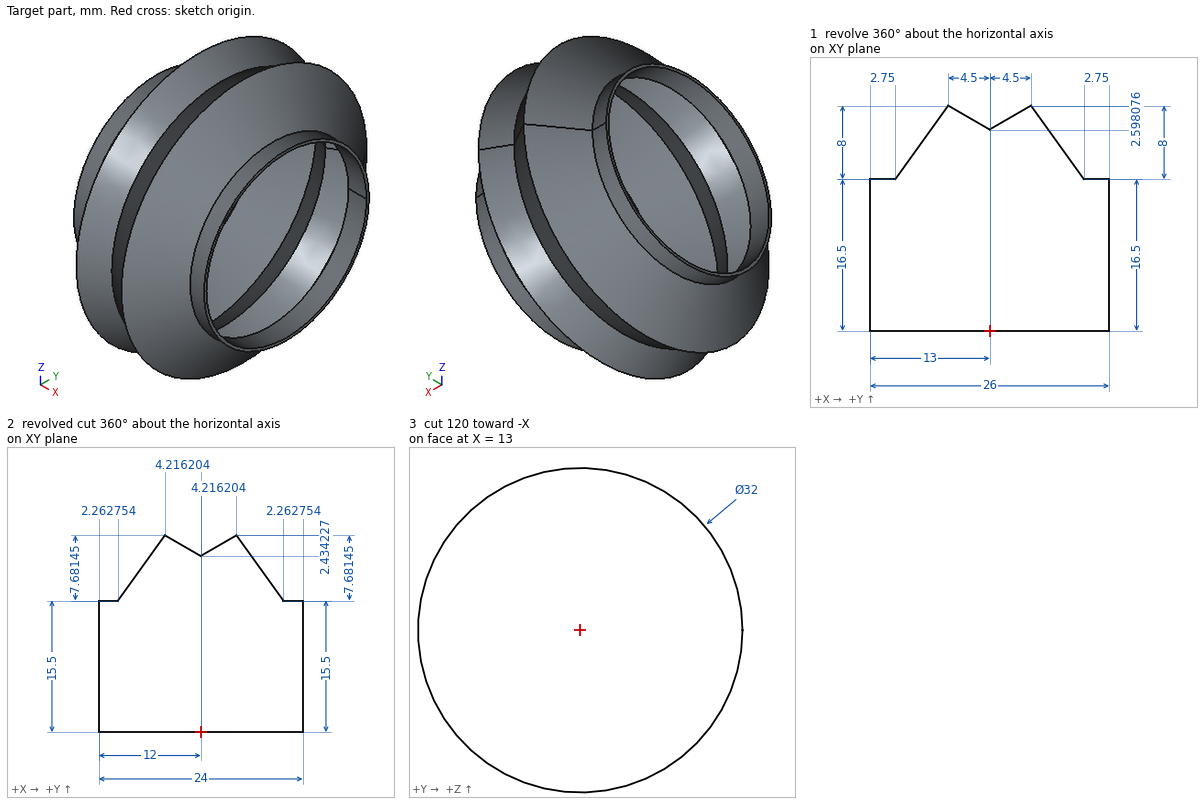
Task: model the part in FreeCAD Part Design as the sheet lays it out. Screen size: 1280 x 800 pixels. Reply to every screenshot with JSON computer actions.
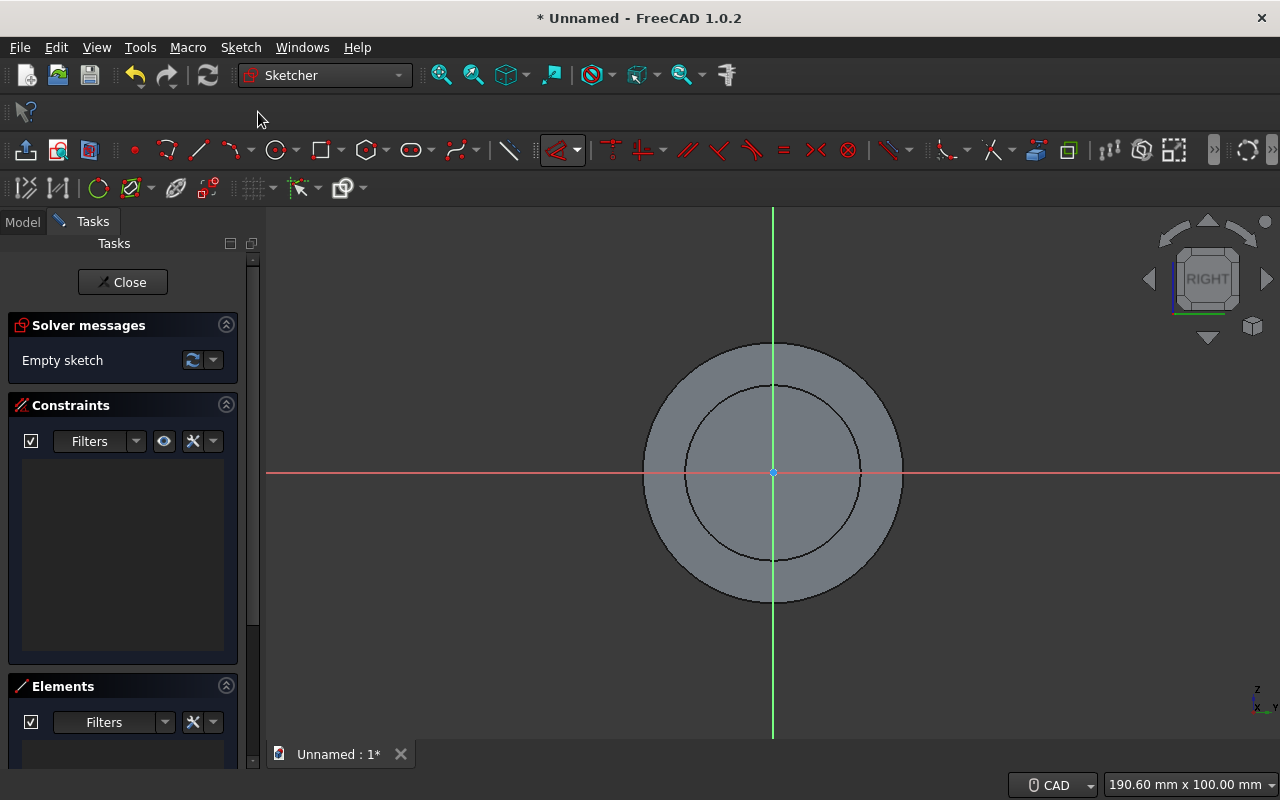
{"action": "scroll", "coordinate": [856, 473], "scroll_direction": "up", "scroll_amount": 3}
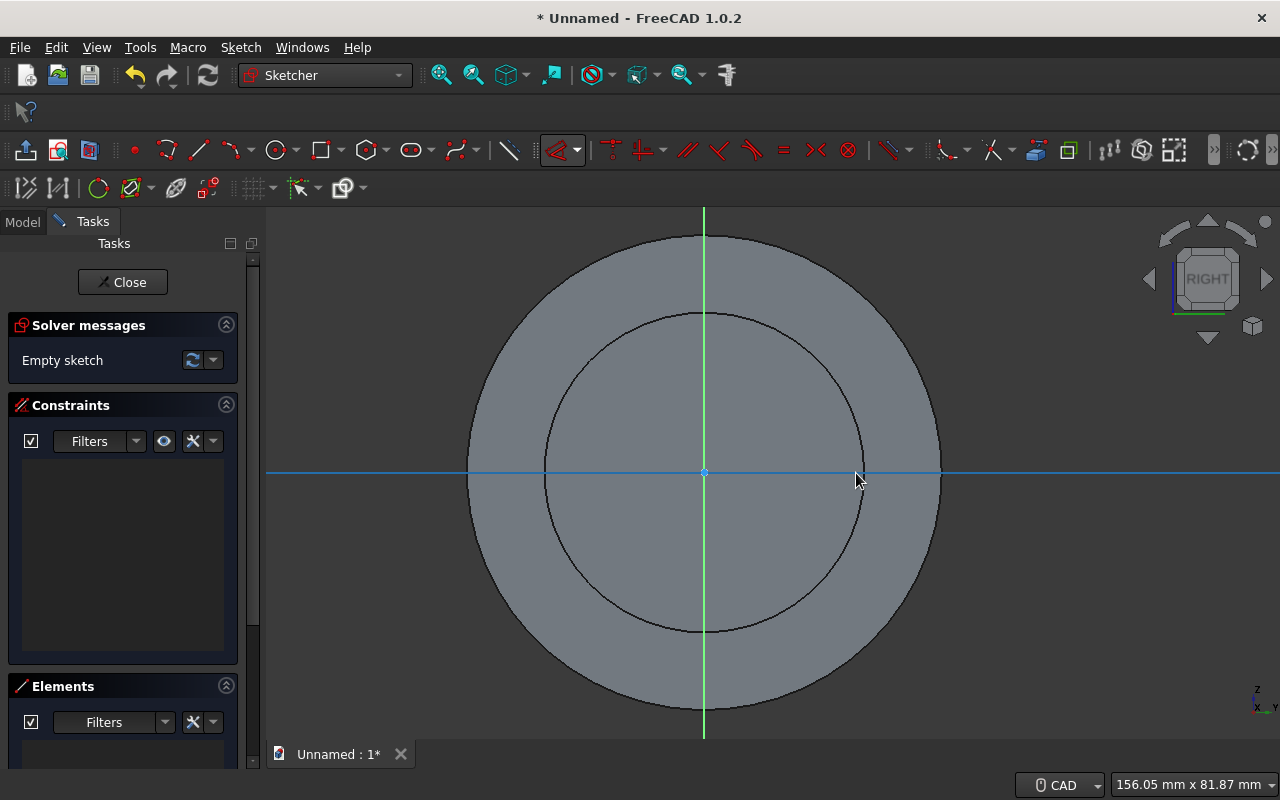
{"action": "left_click", "coordinate": [276, 150]}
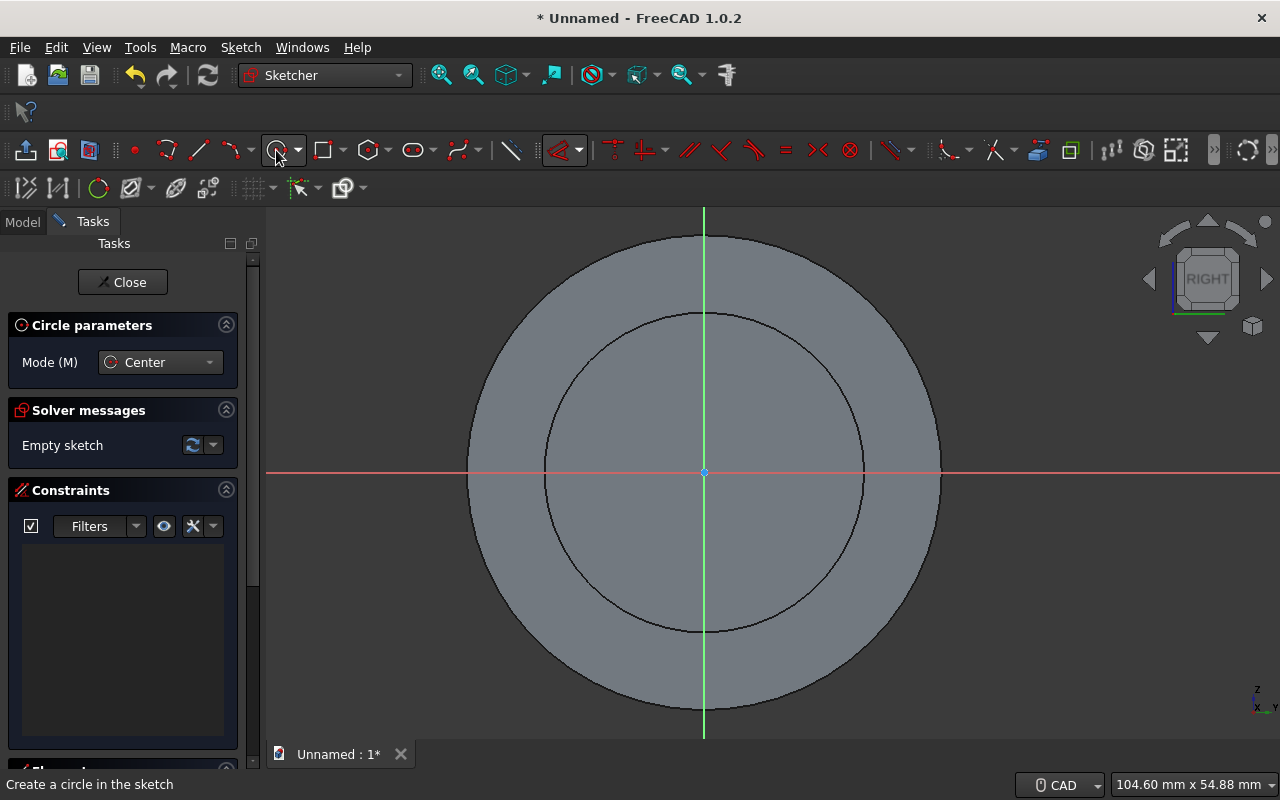
{"action": "left_click", "coordinate": [704, 473]}
{"action": "mouse_move", "coordinate": [814, 363]}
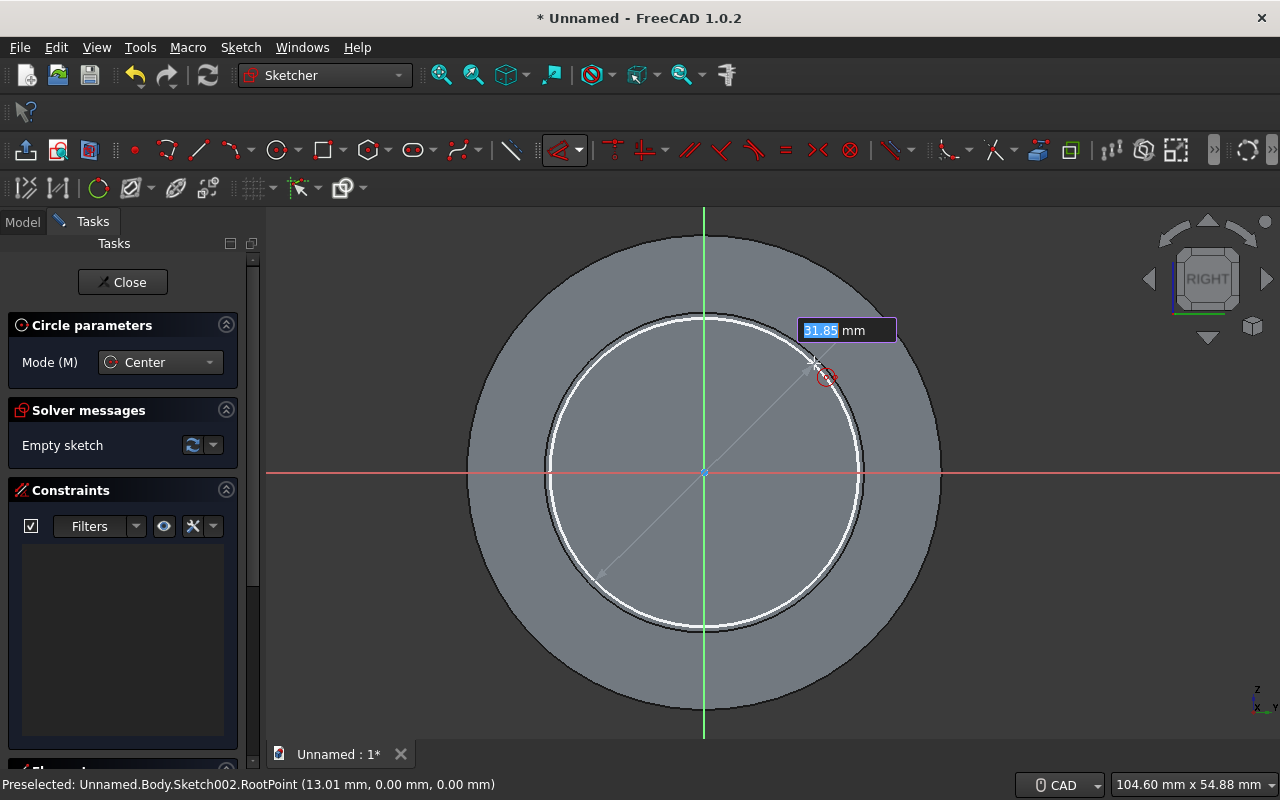
{"action": "type", "text": "32"}
{"action": "key", "text": "Return"}
{"action": "key", "text": "Escape"}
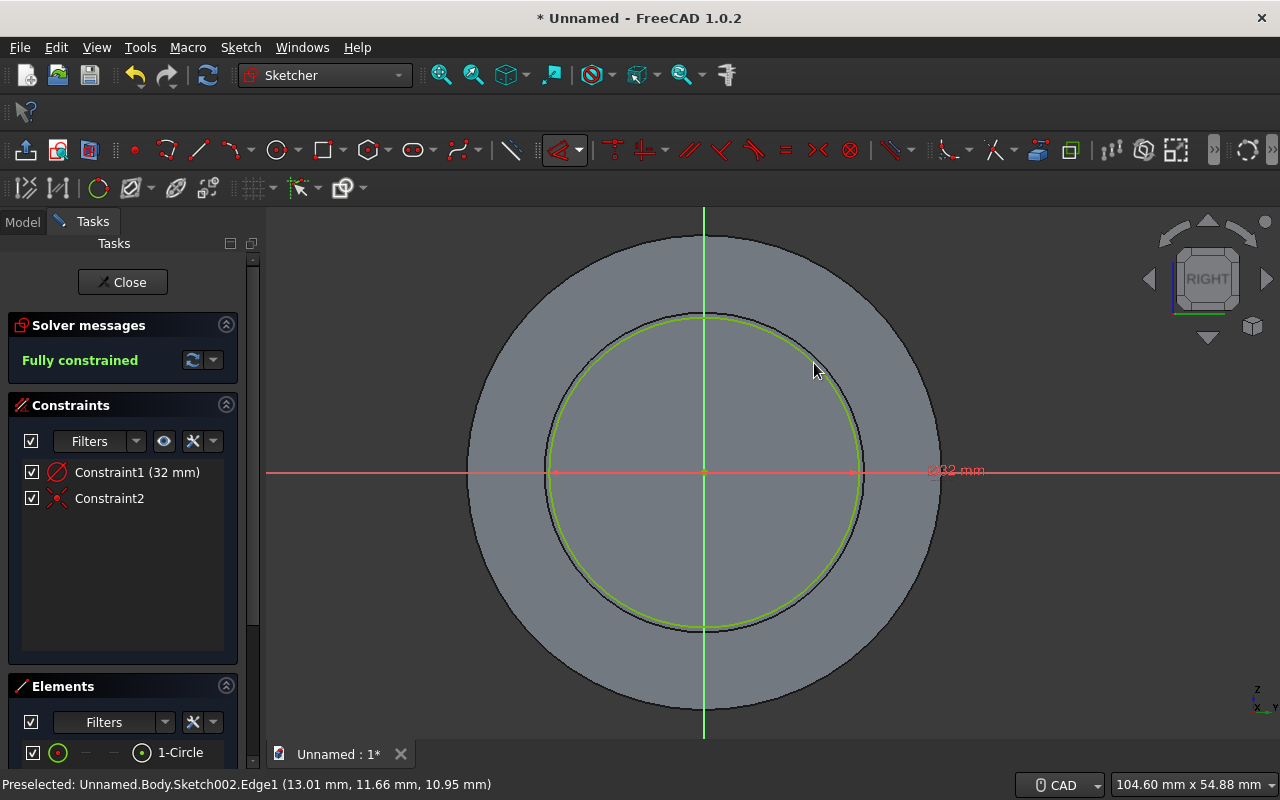
{"action": "left_click", "coordinate": [123, 282]}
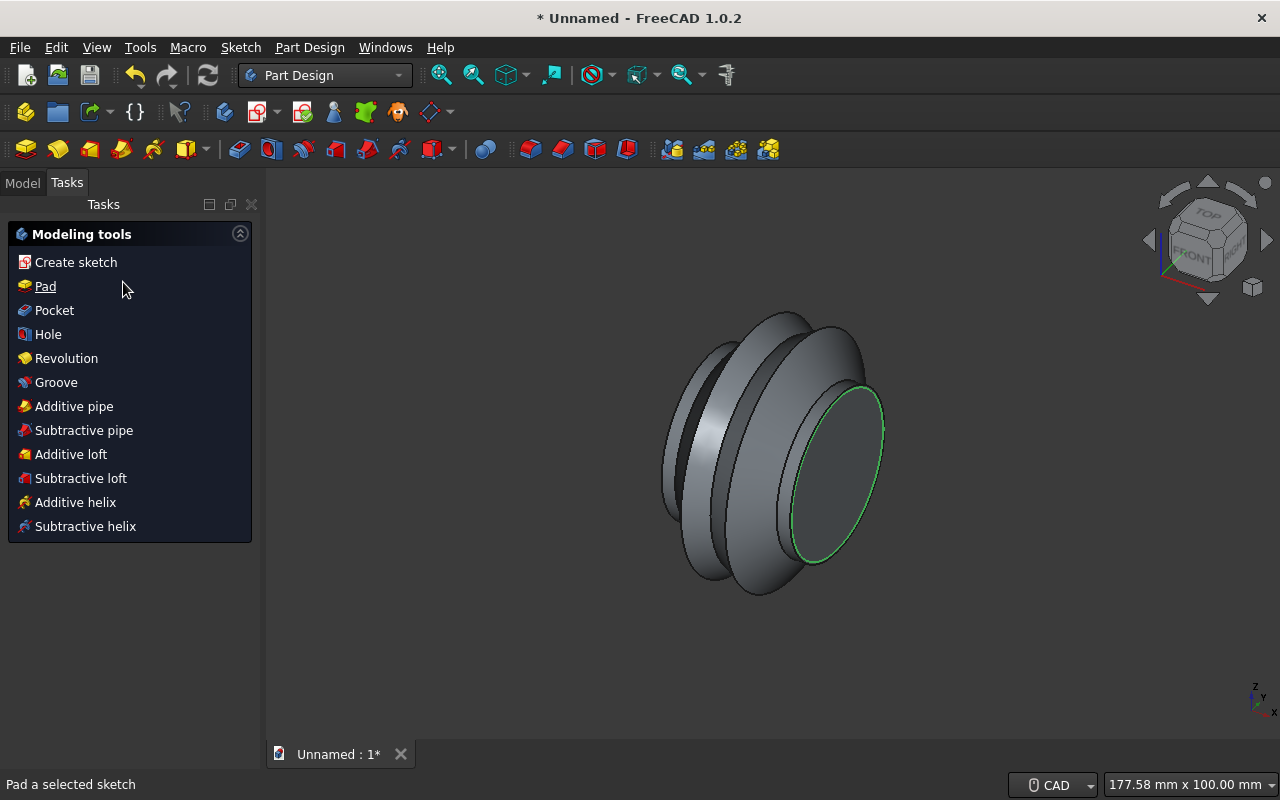
{"action": "left_click", "coordinate": [240, 150]}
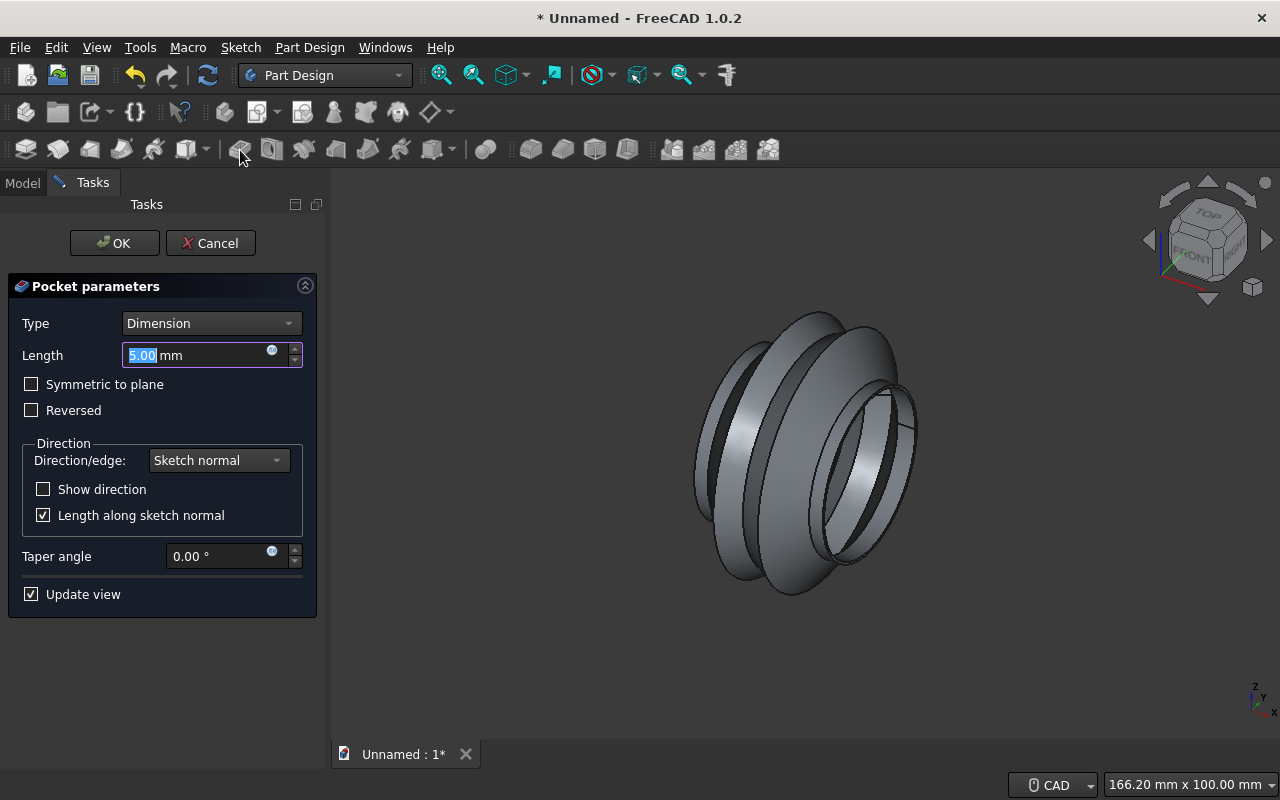
{"action": "type", "text": "120"}
{"action": "key", "text": "Tab"}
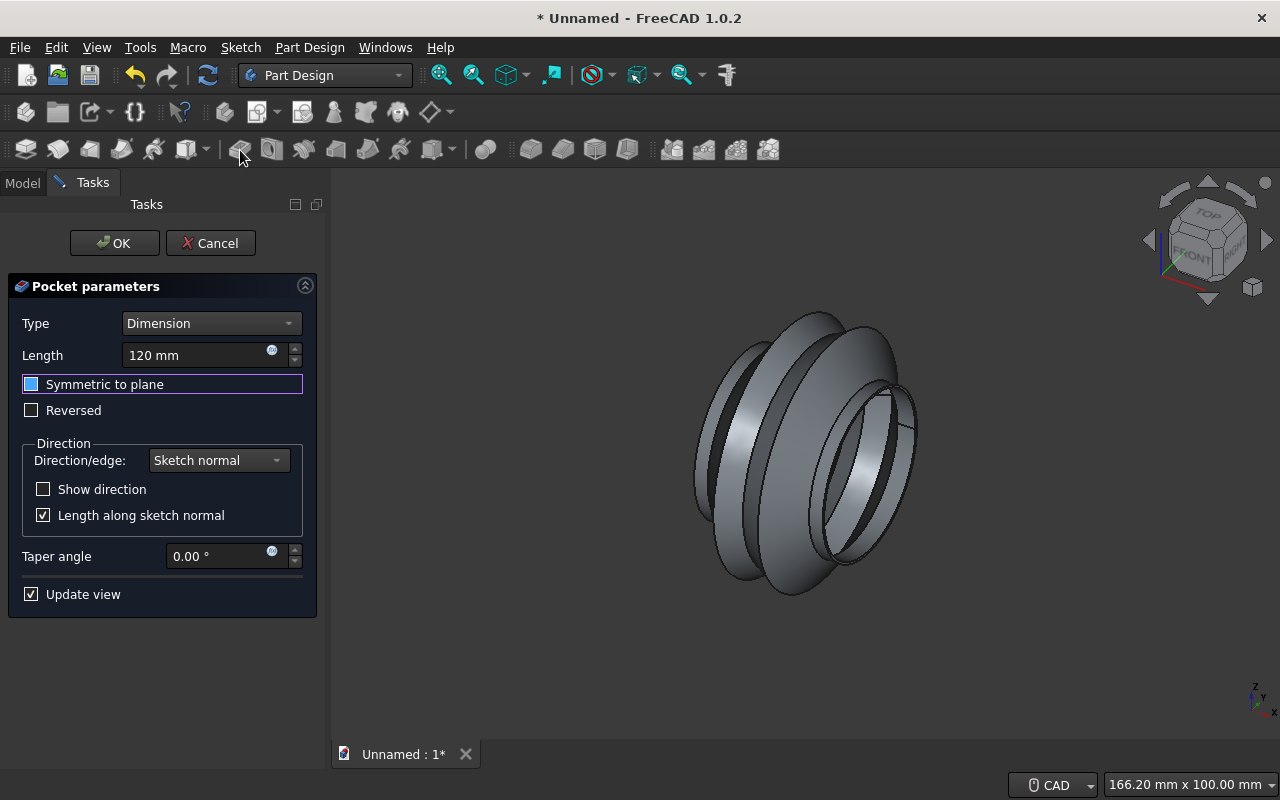
{"action": "left_click", "coordinate": [115, 243]}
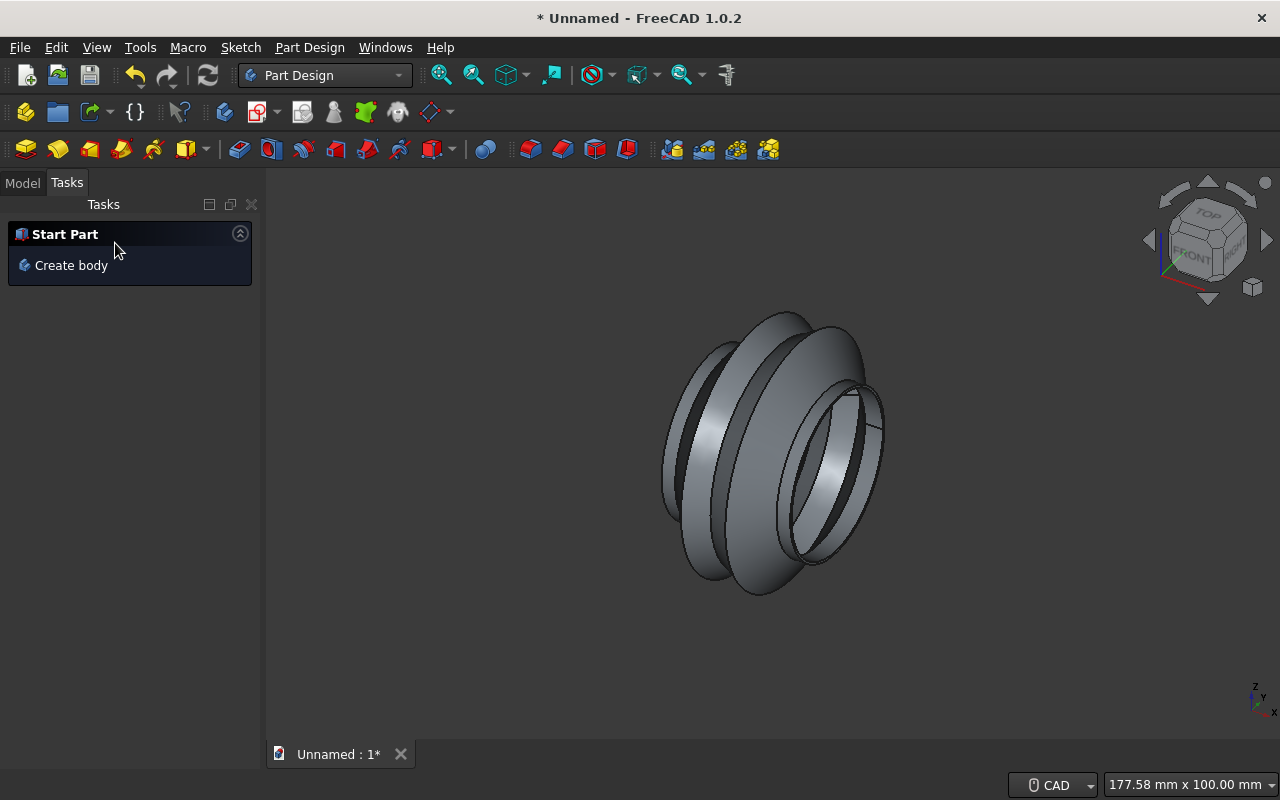
{"action": "key", "text": "0"}